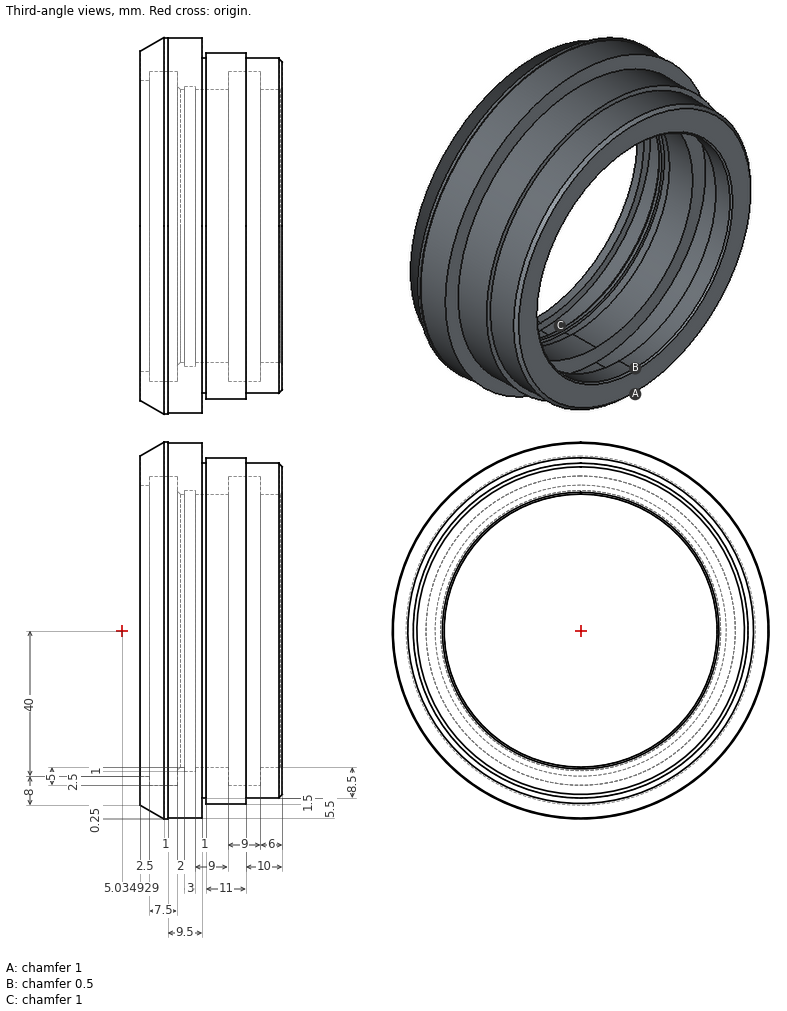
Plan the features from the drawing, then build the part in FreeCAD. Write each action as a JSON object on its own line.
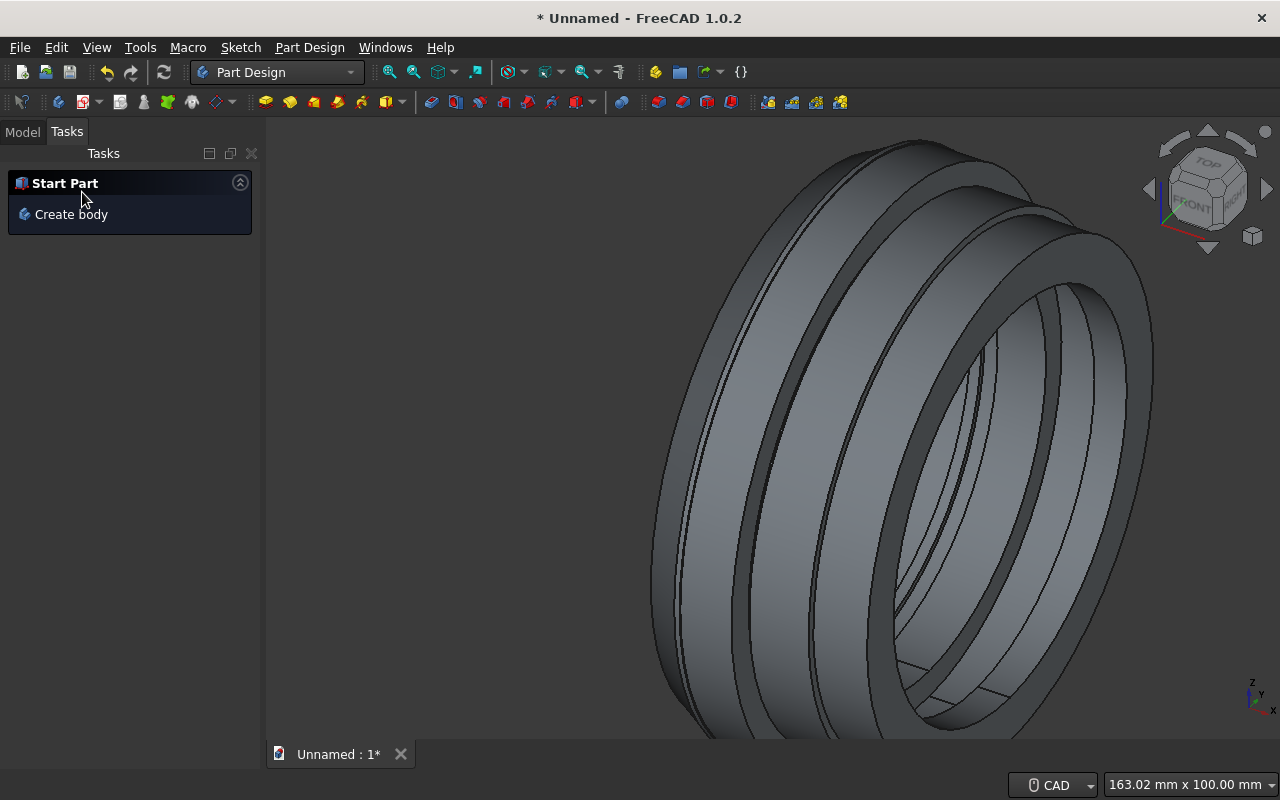
{"action": "key", "text": "v f"}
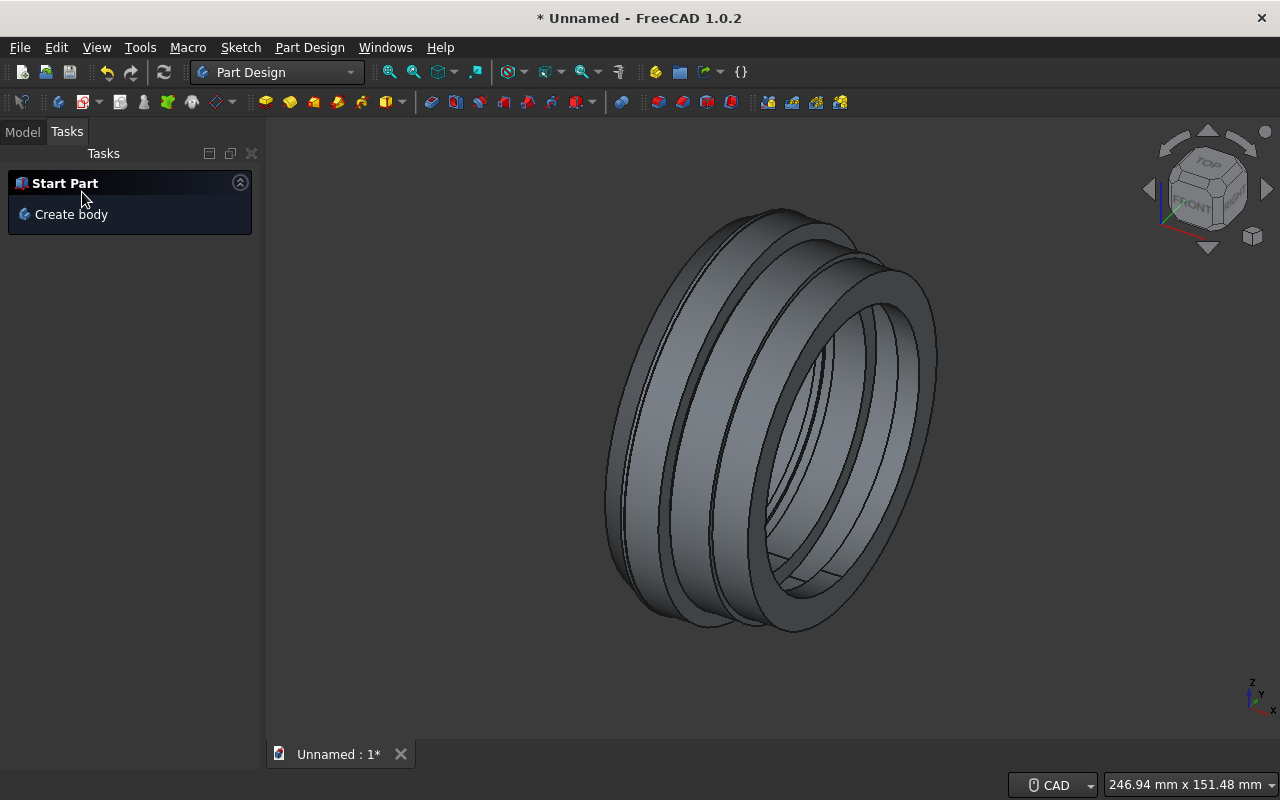
{"action": "left_click", "coordinate": [842, 295]}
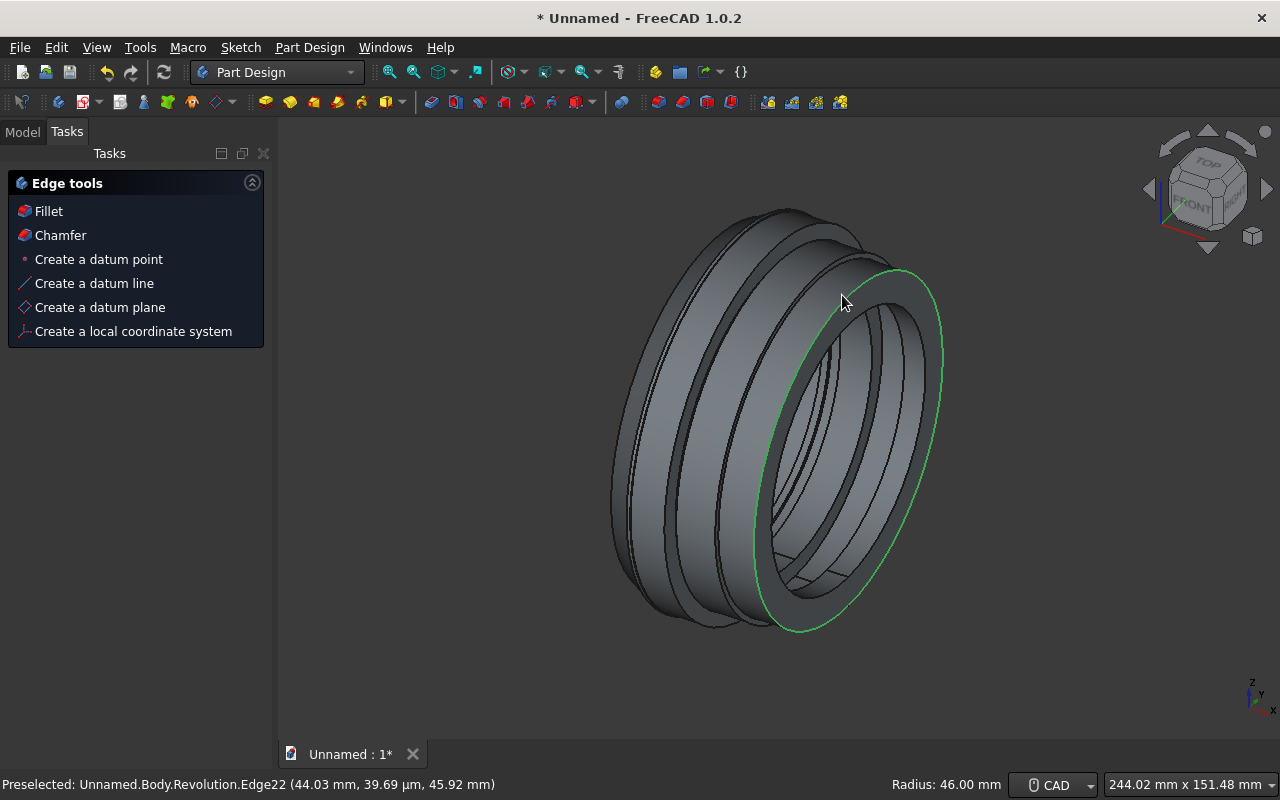
{"action": "left_click", "coordinate": [684, 102]}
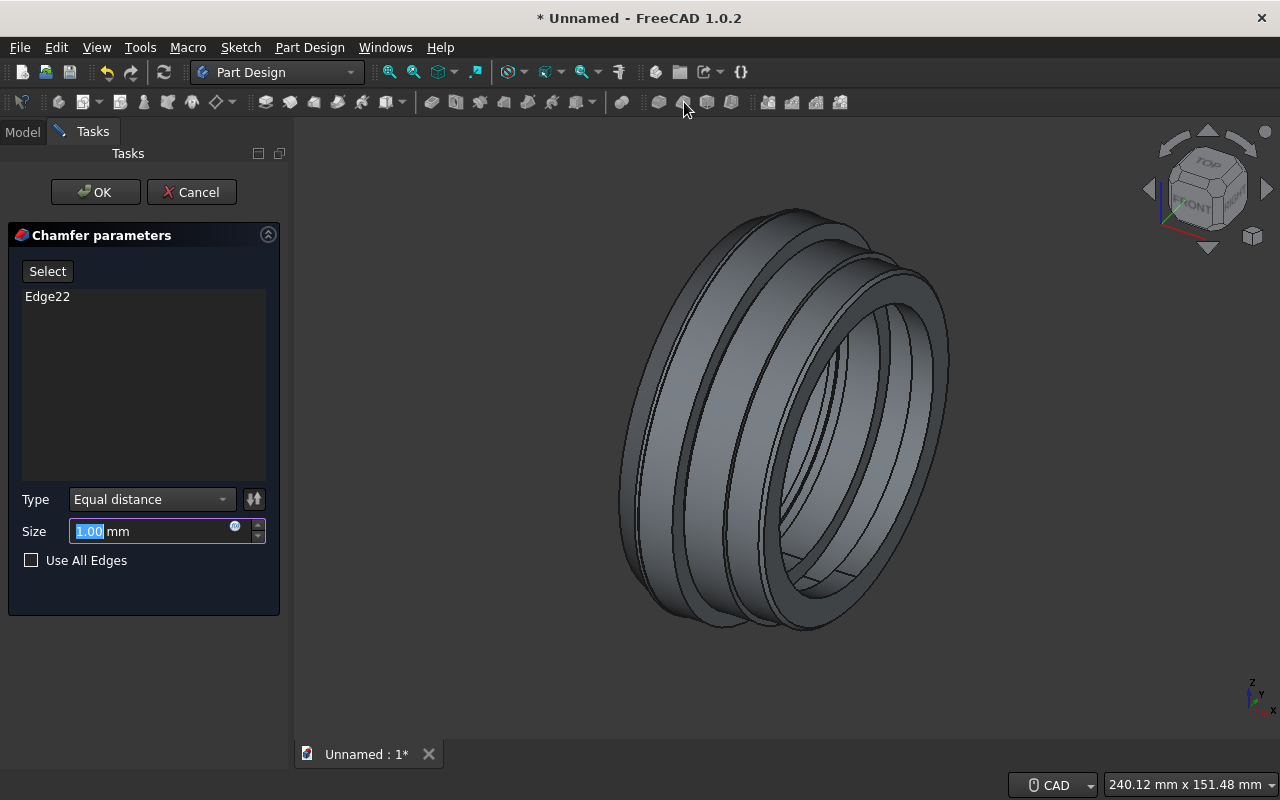
{"action": "type", "text": "1"}
{"action": "key", "text": "Tab"}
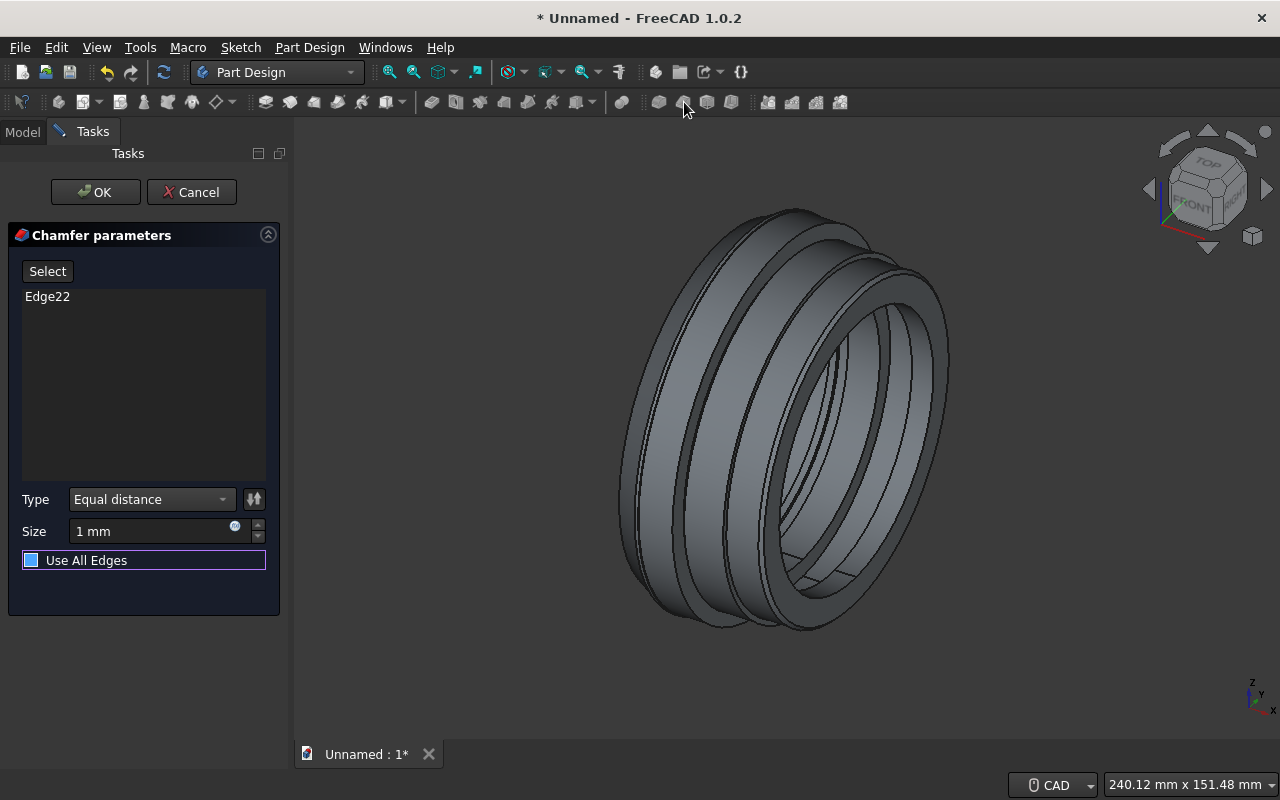
{"action": "left_click", "coordinate": [96, 192]}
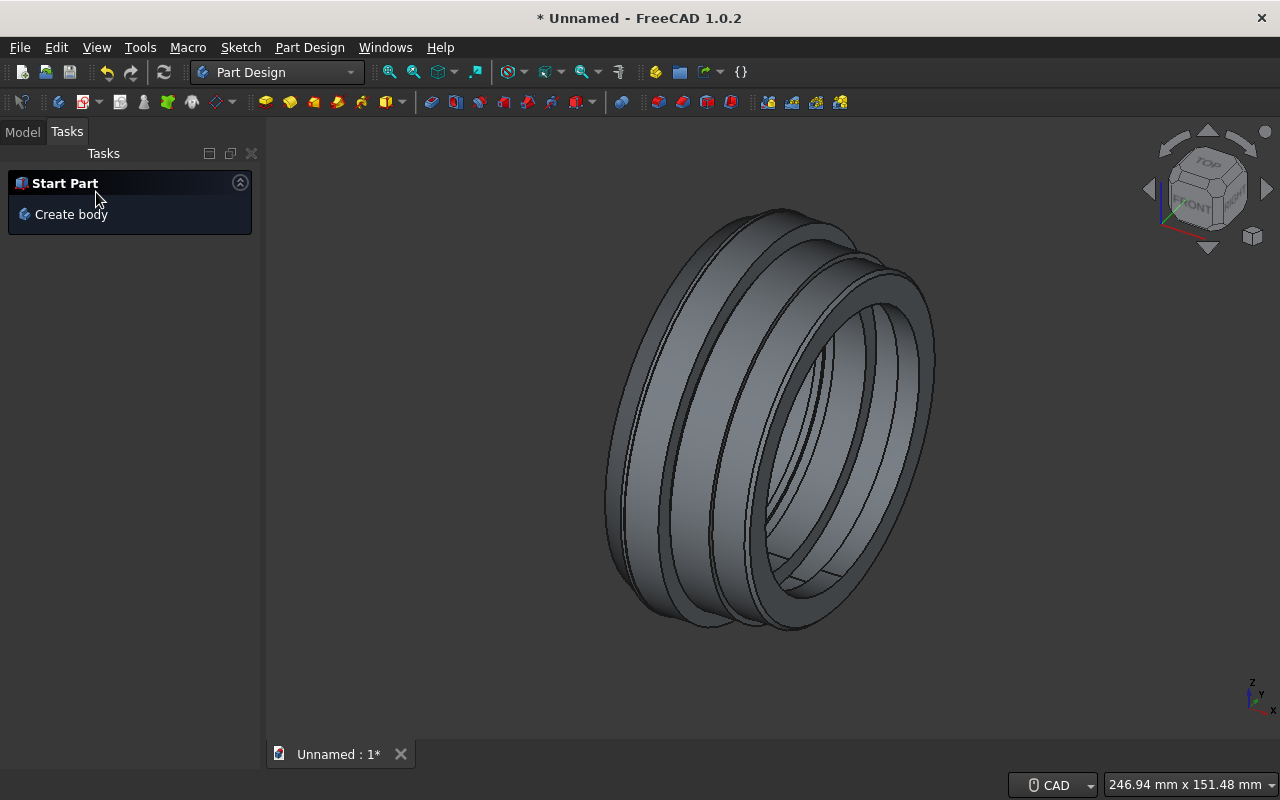
{"action": "left_click", "coordinate": [916, 338]}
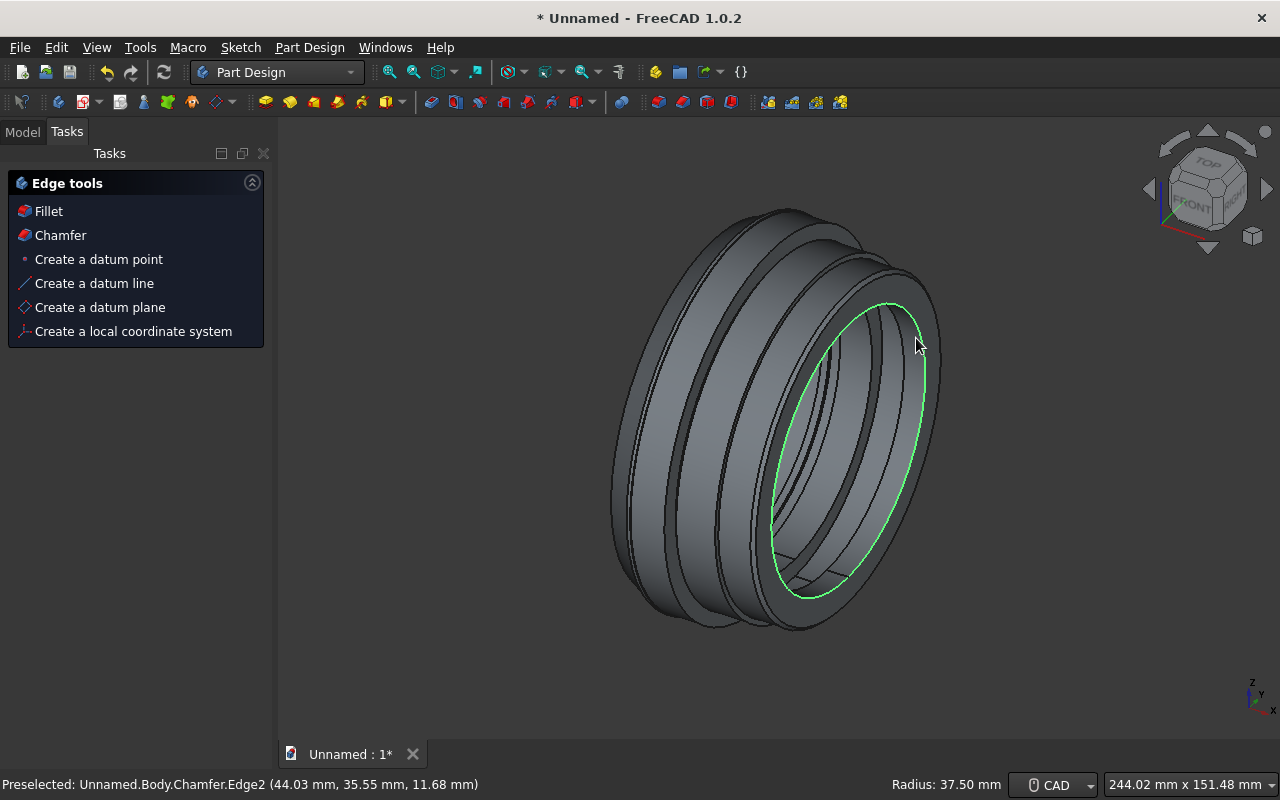
{"action": "left_click", "coordinate": [684, 102]}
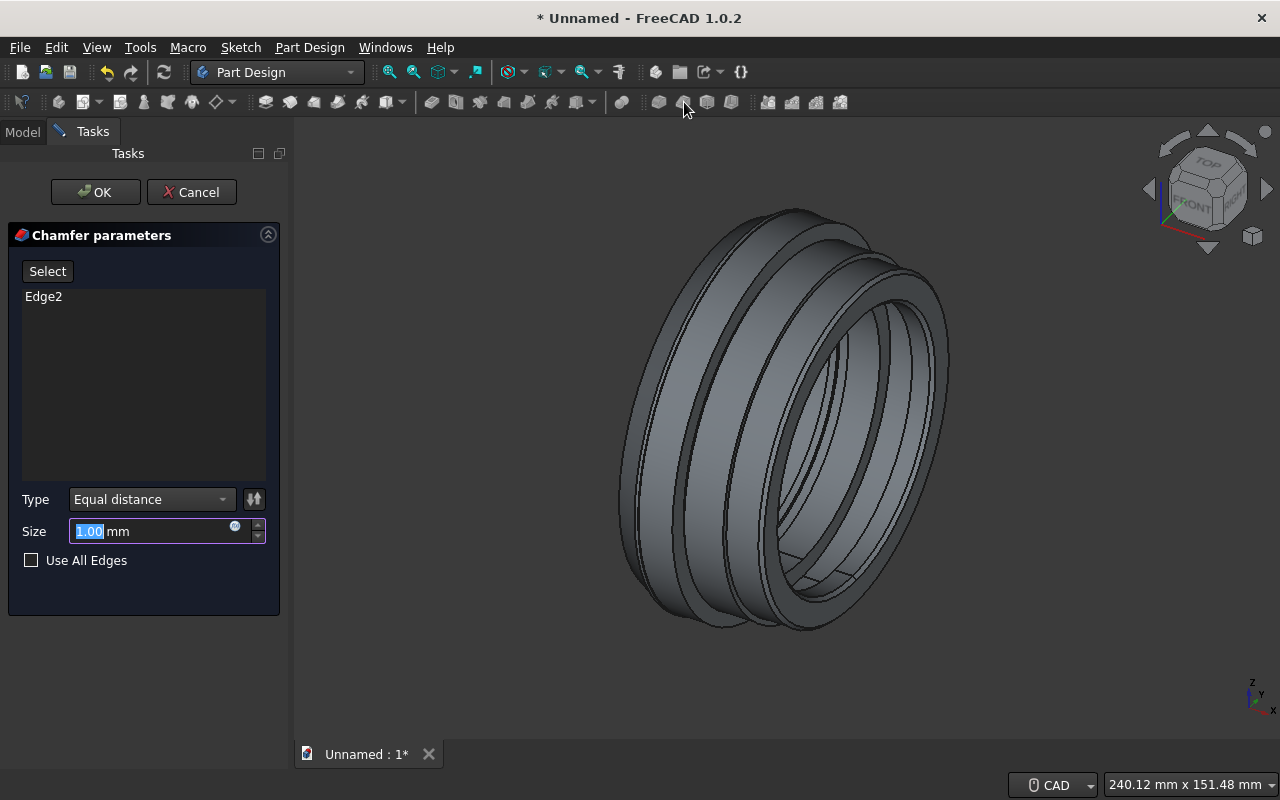
{"action": "type", "text": "0.5"}
{"action": "key", "text": "Tab"}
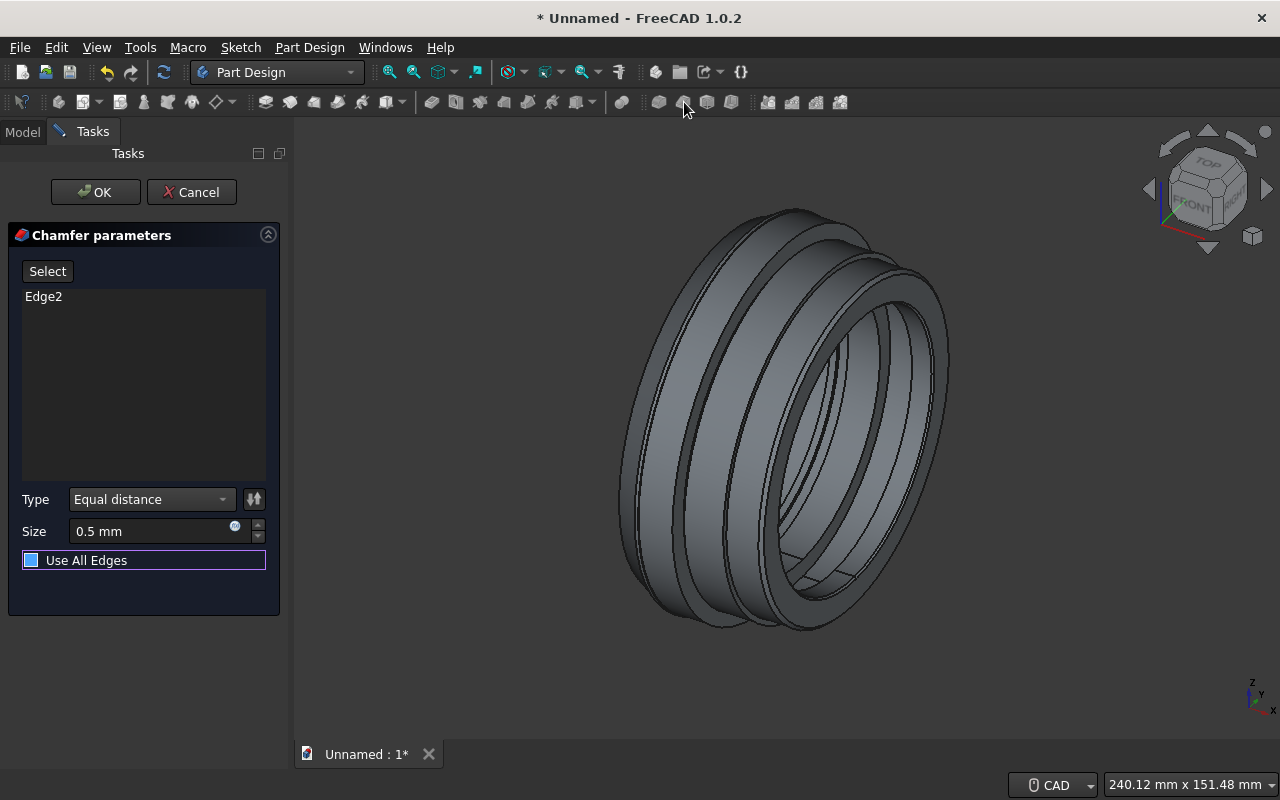
{"action": "left_click", "coordinate": [96, 192]}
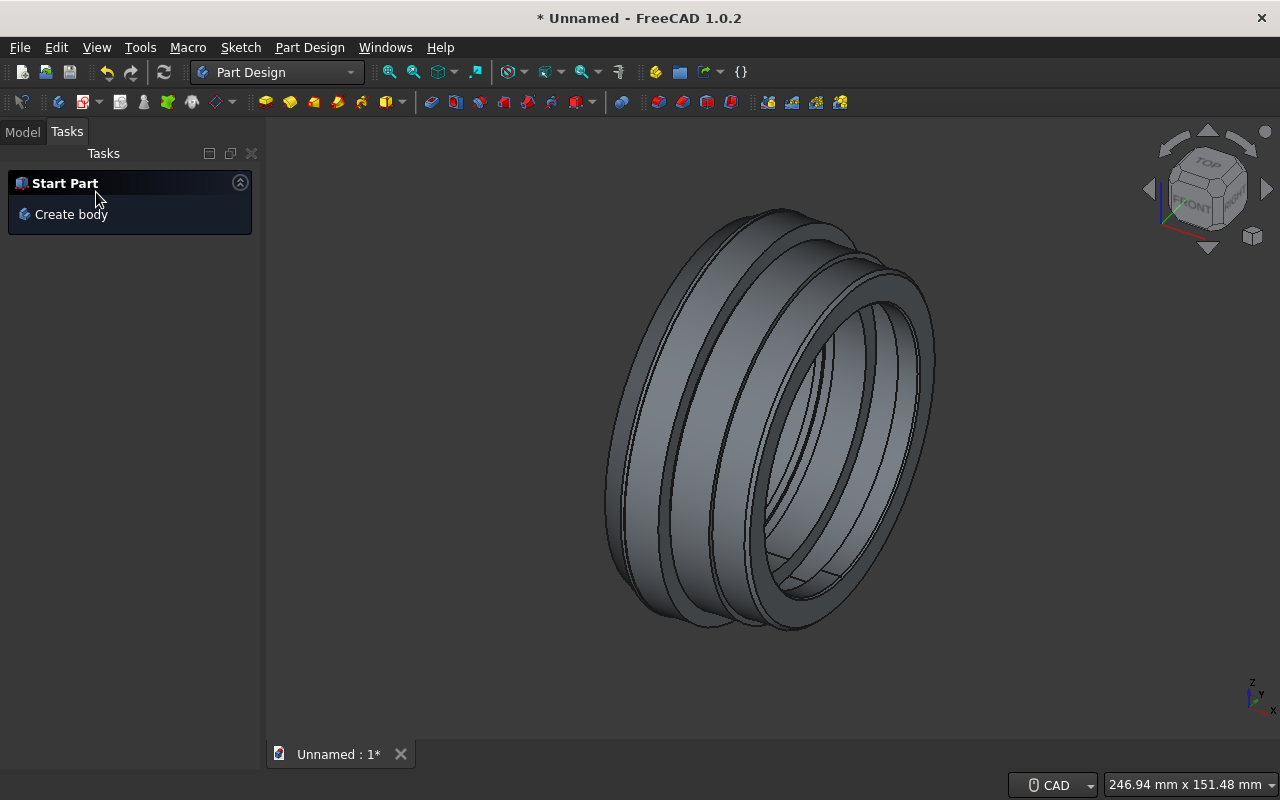
{"action": "key", "text": "0"}